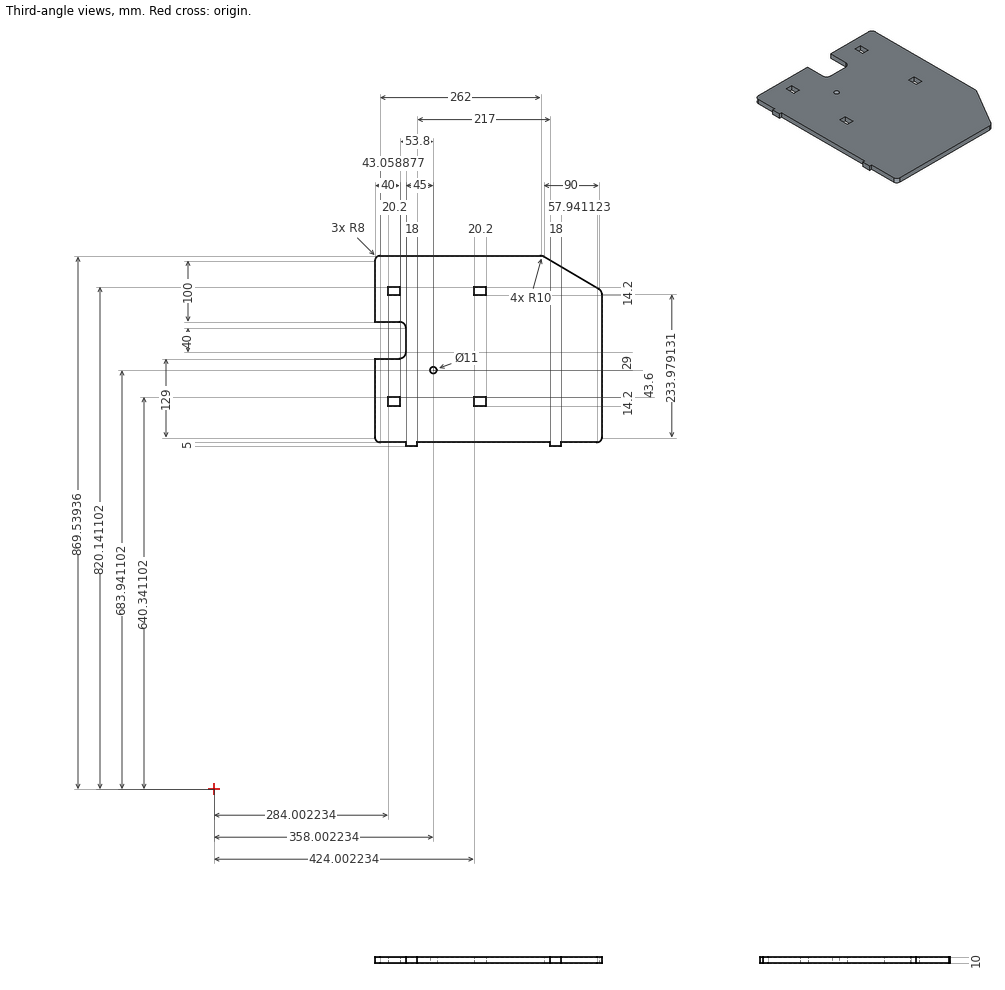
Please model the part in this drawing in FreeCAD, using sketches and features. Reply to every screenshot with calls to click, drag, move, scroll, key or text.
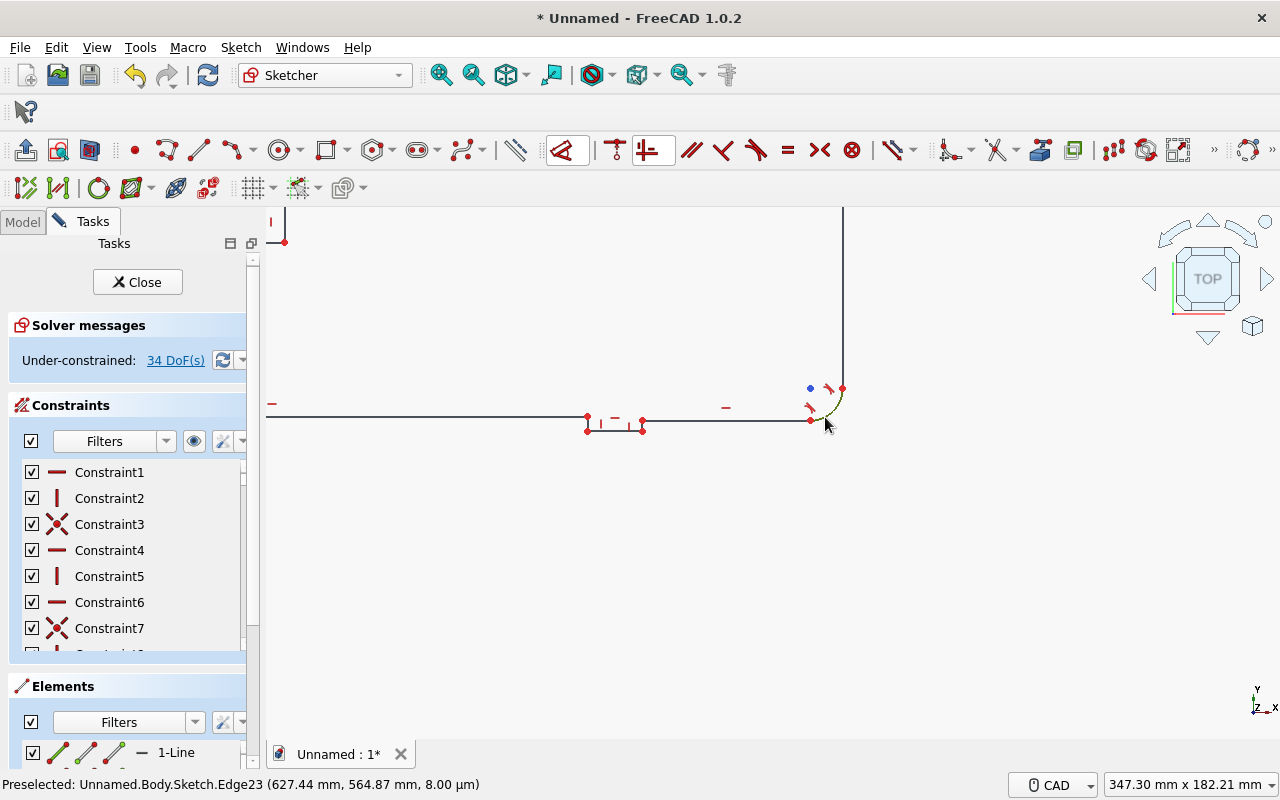
key(e)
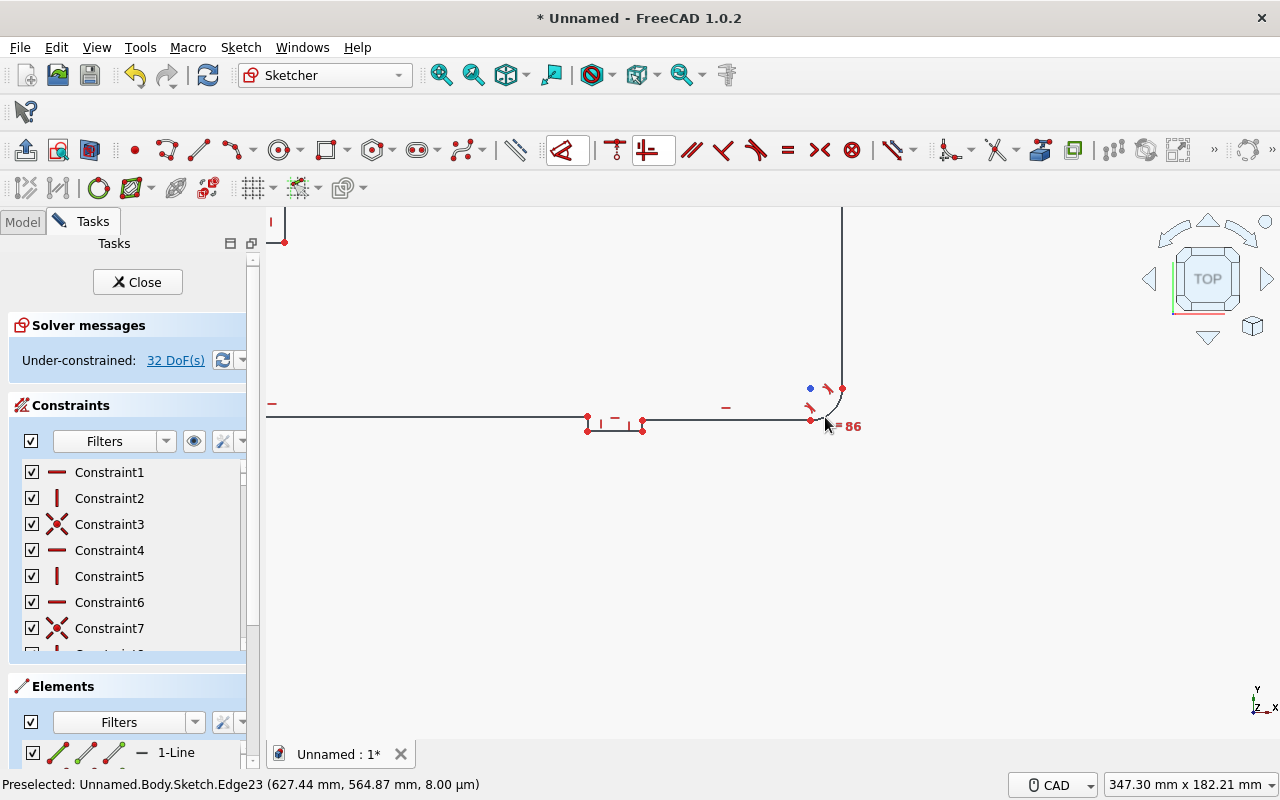
click(562, 150)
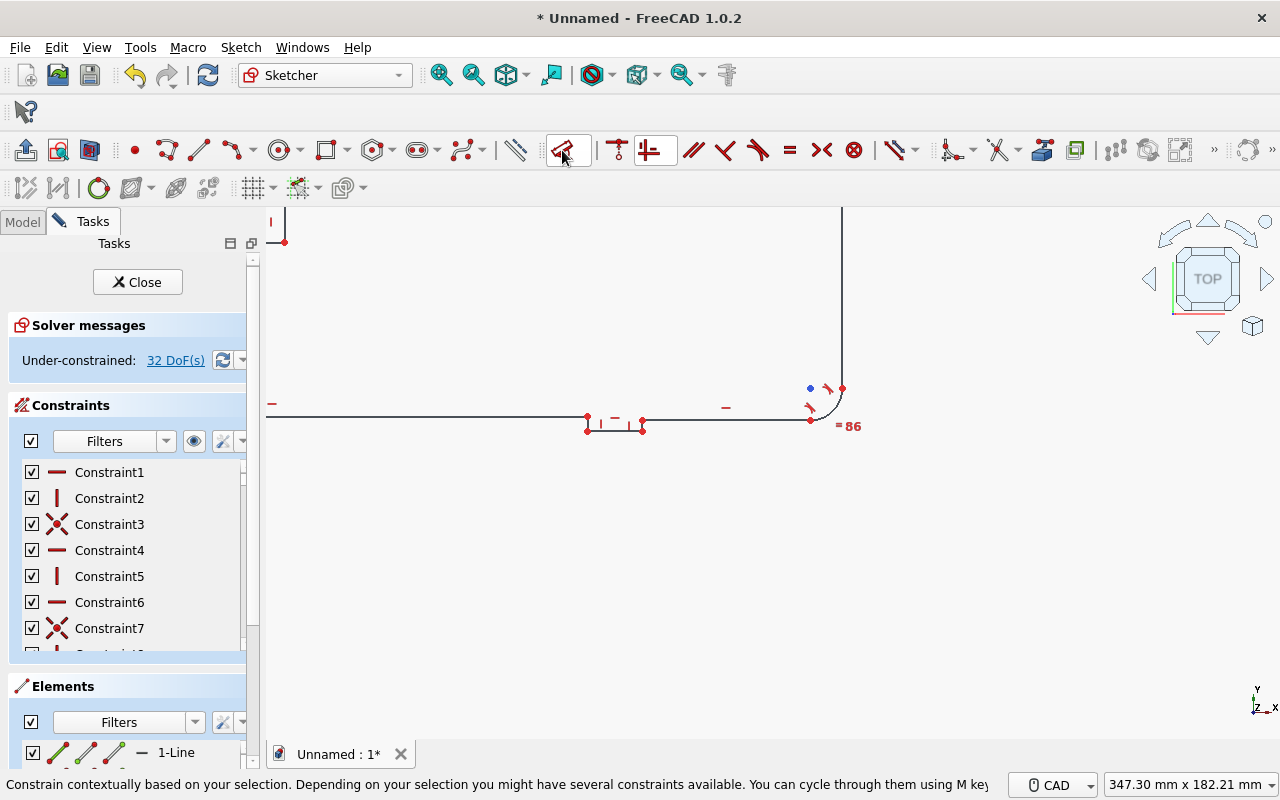
scroll(828, 422, down, 10)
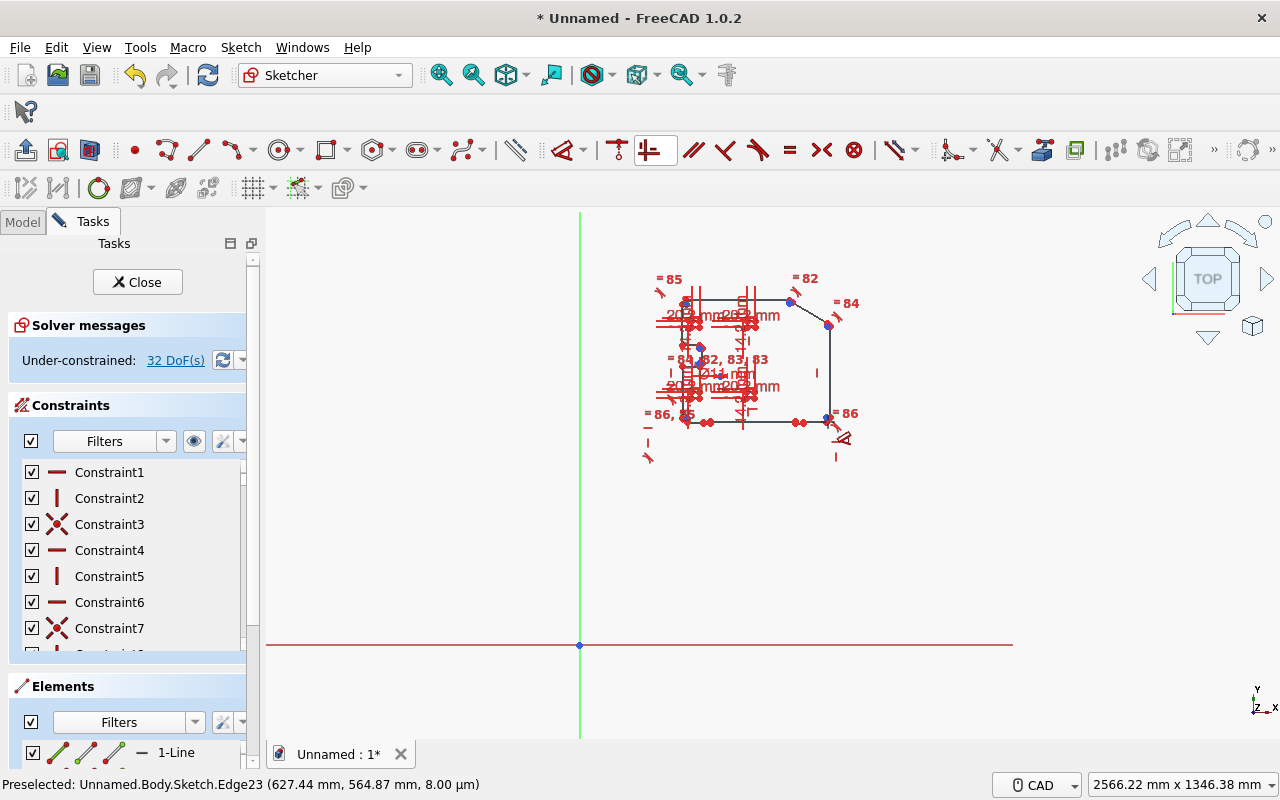
scroll(791, 301, up, 12)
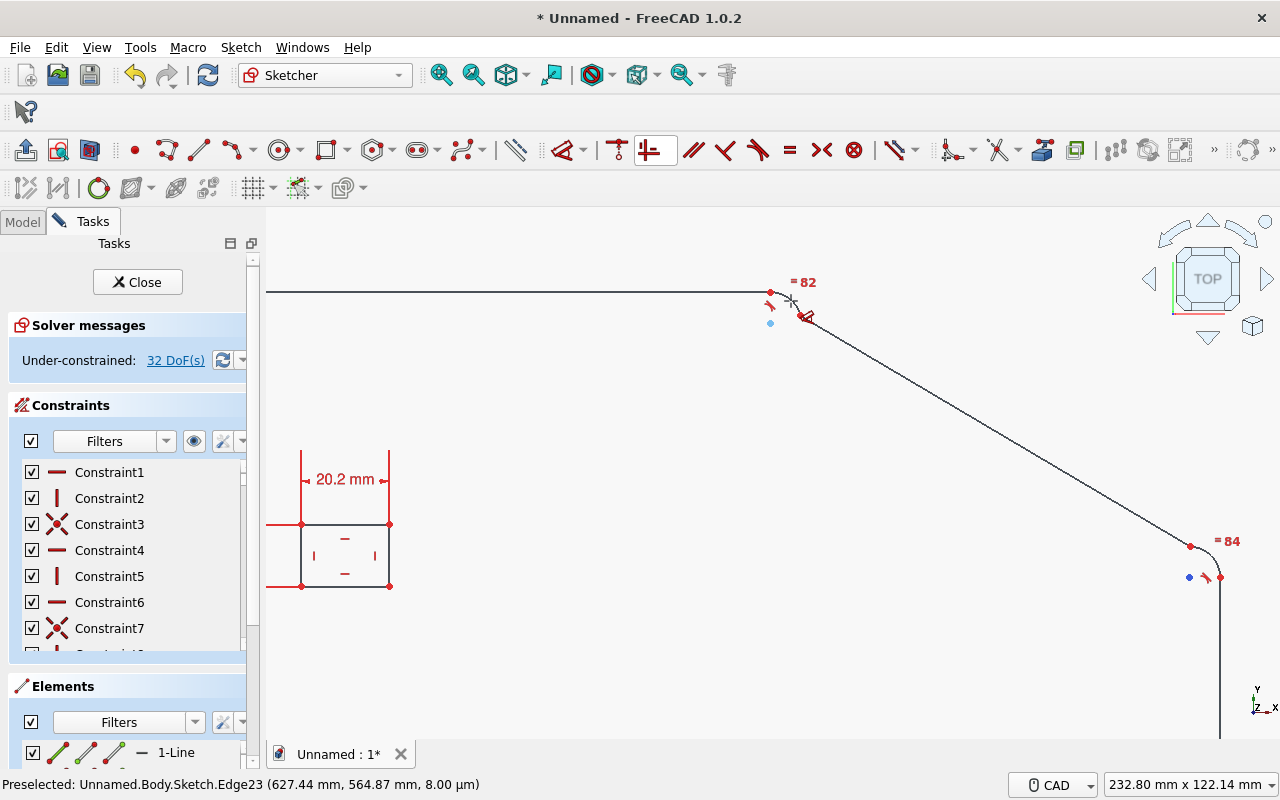
click(790, 299)
click(810, 274)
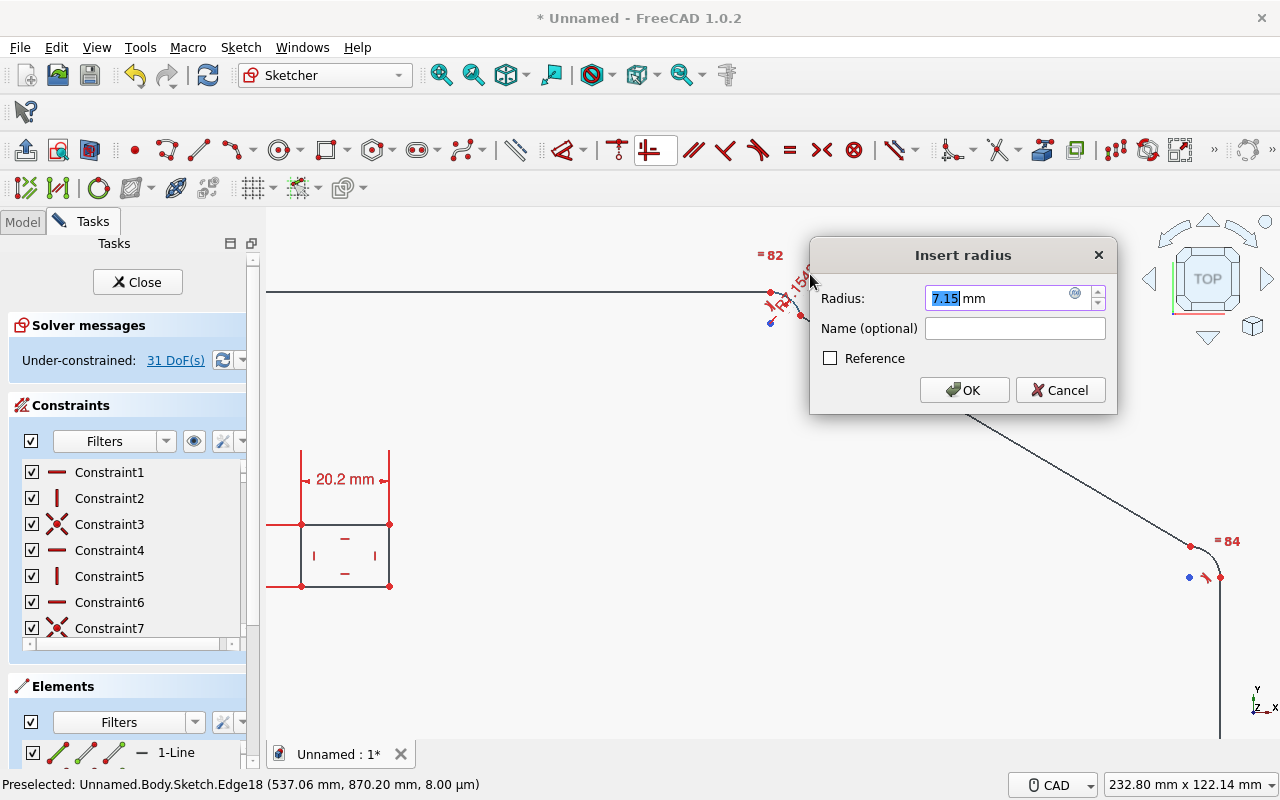
text(10)
key(Return)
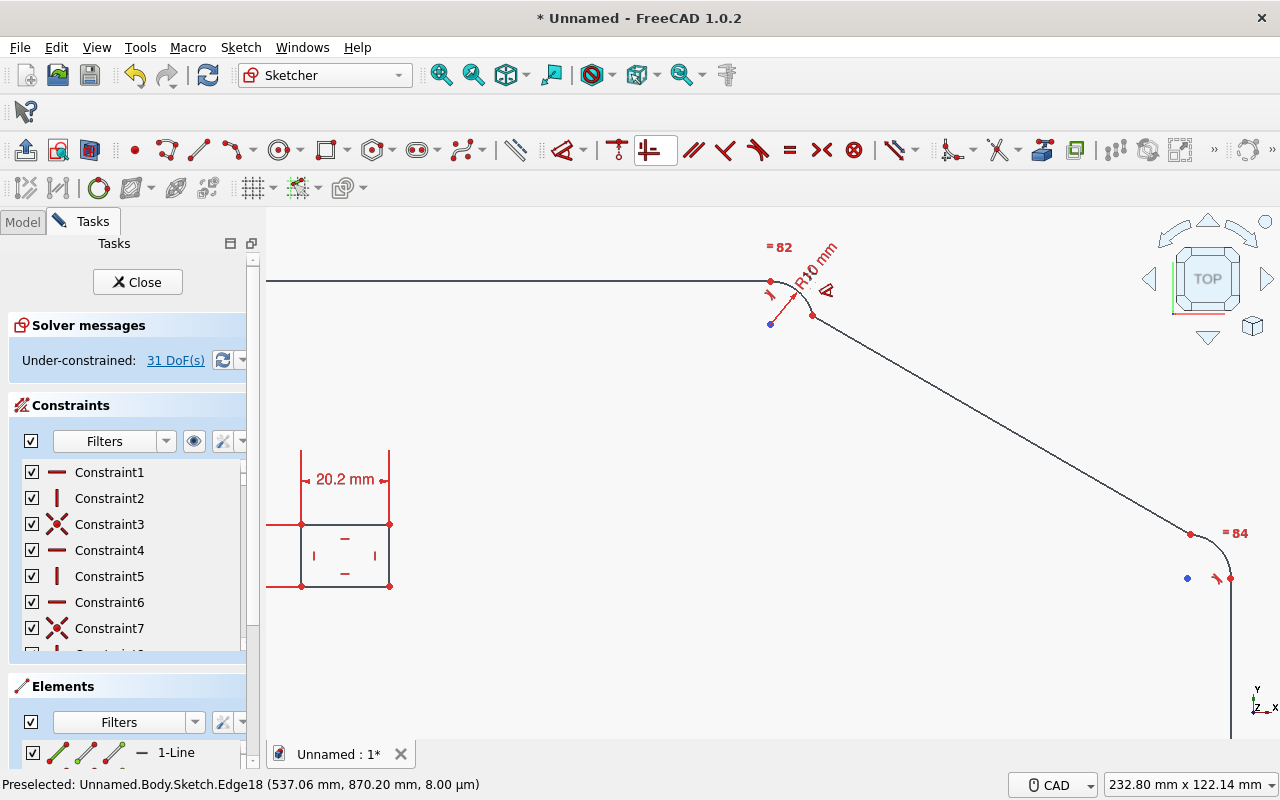
scroll(791, 301, down, 12)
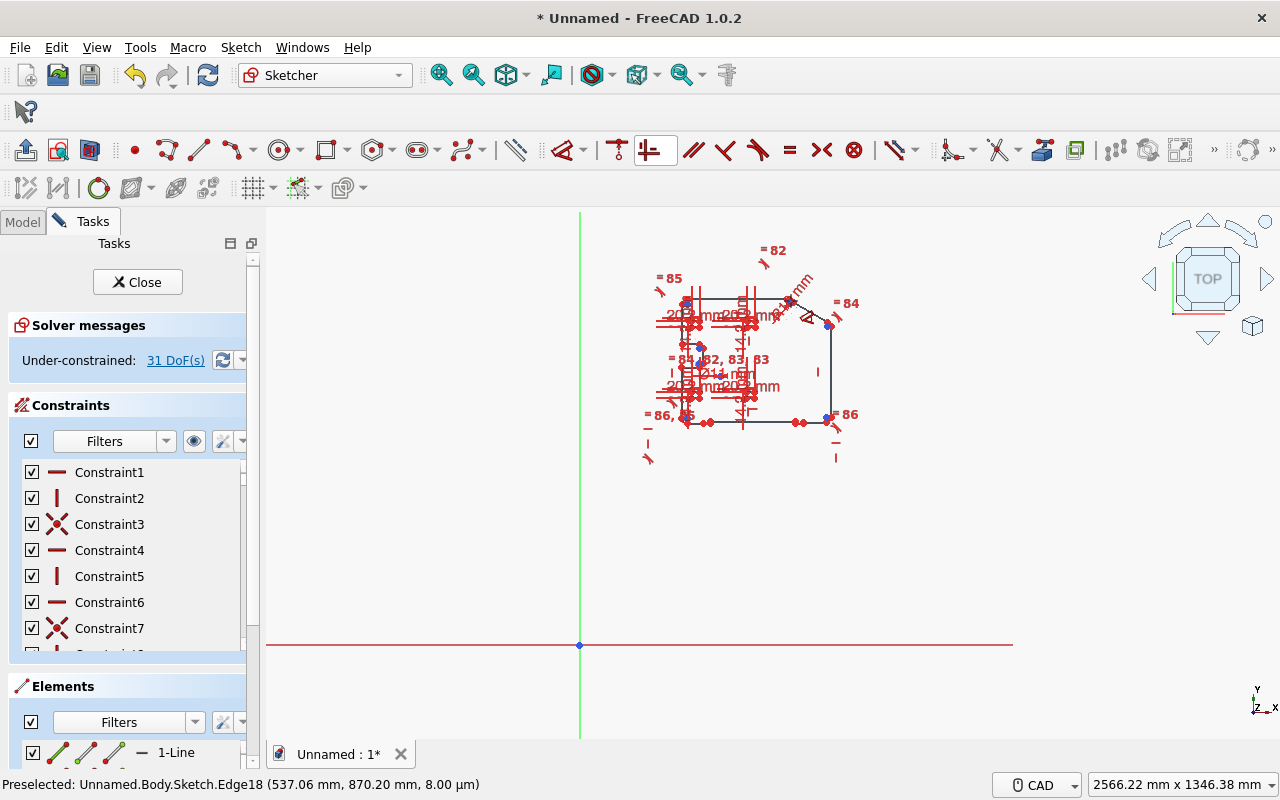
scroll(685, 300, up, 13)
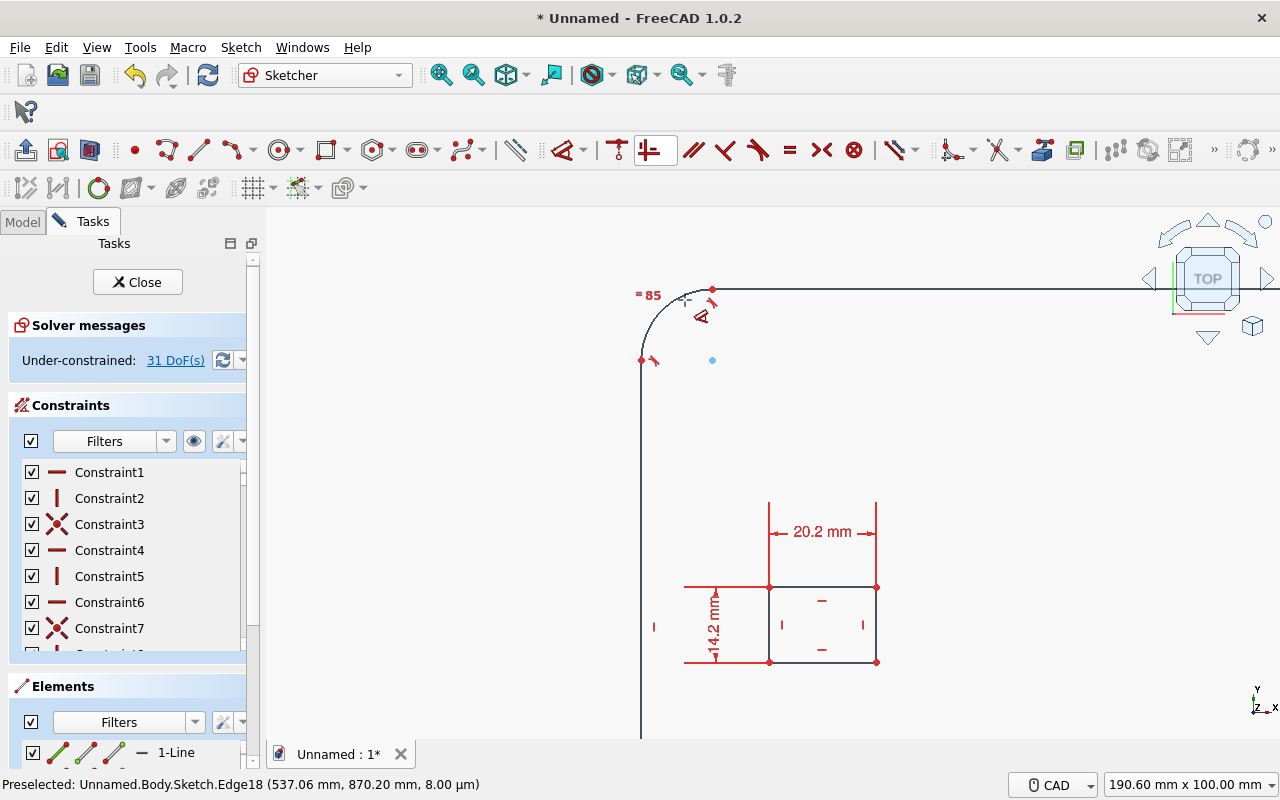
click(680, 297)
click(665, 269)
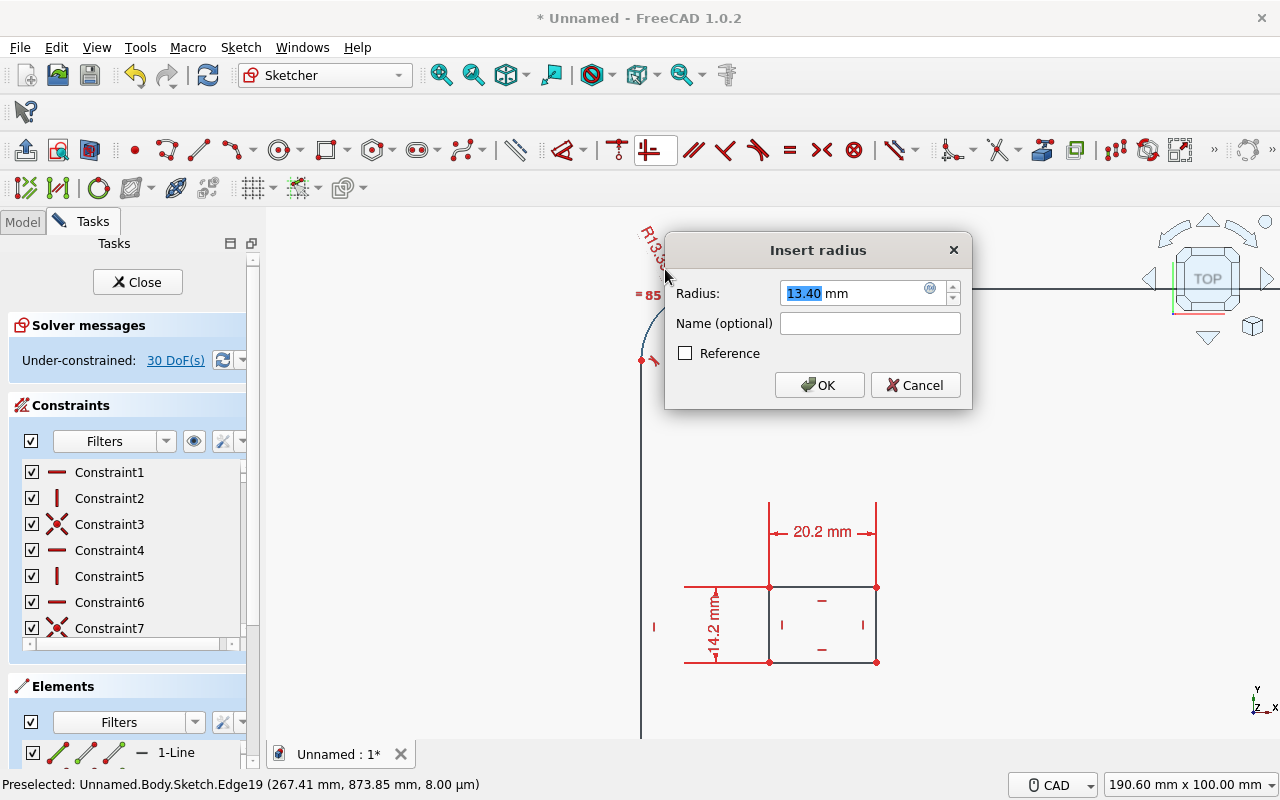
text(8)
key(Return)